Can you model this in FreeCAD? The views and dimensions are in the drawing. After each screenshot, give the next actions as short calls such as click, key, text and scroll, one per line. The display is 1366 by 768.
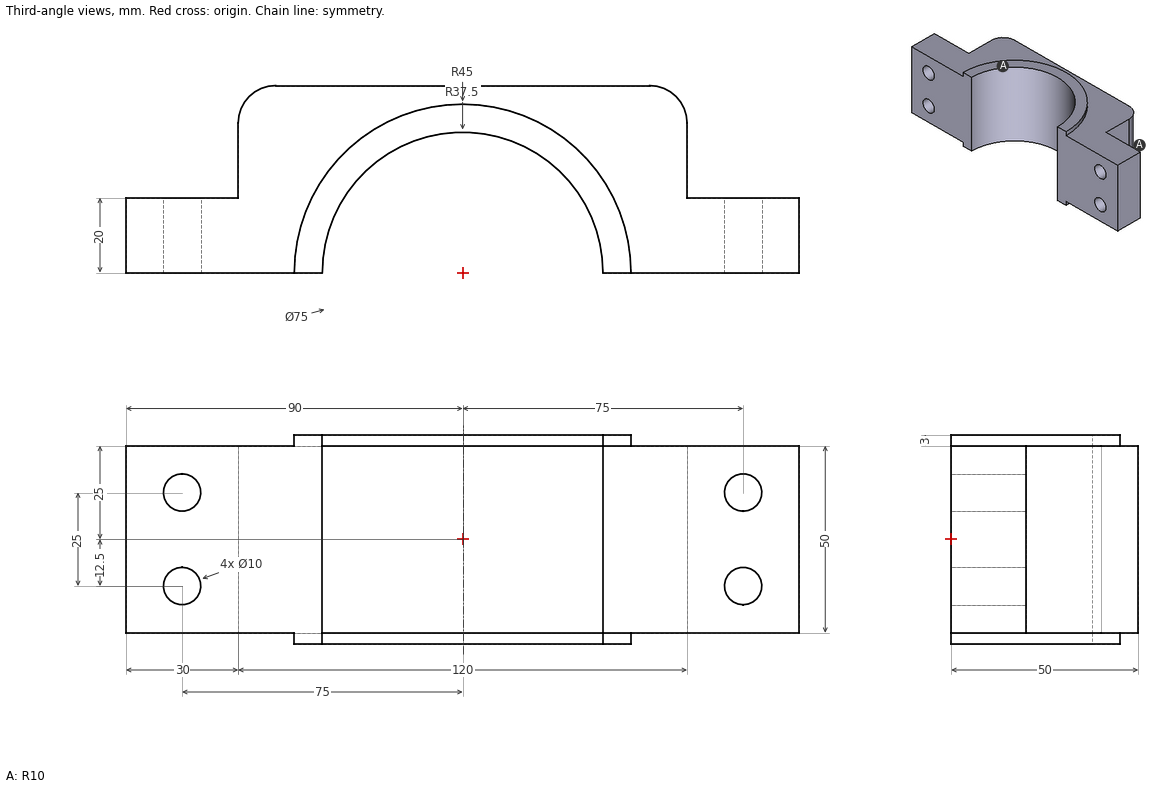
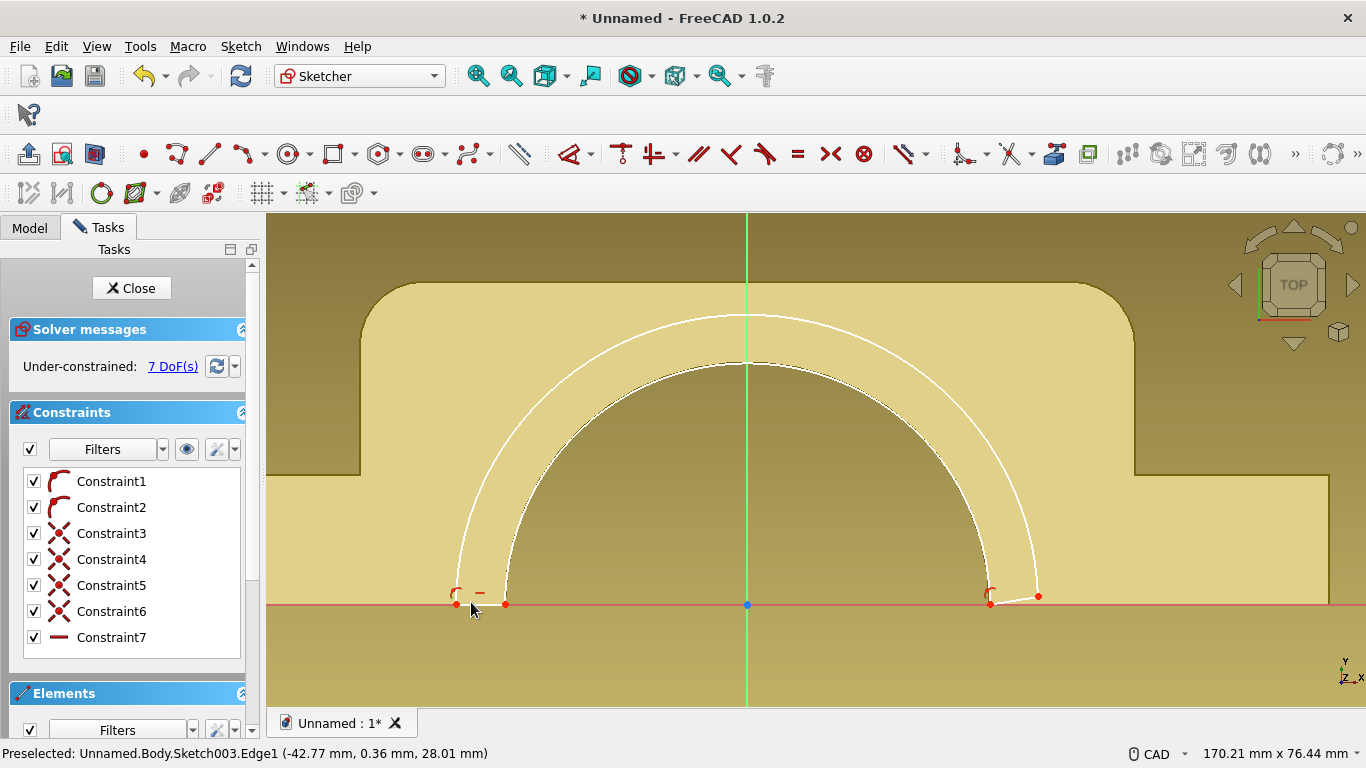
click(1004, 602)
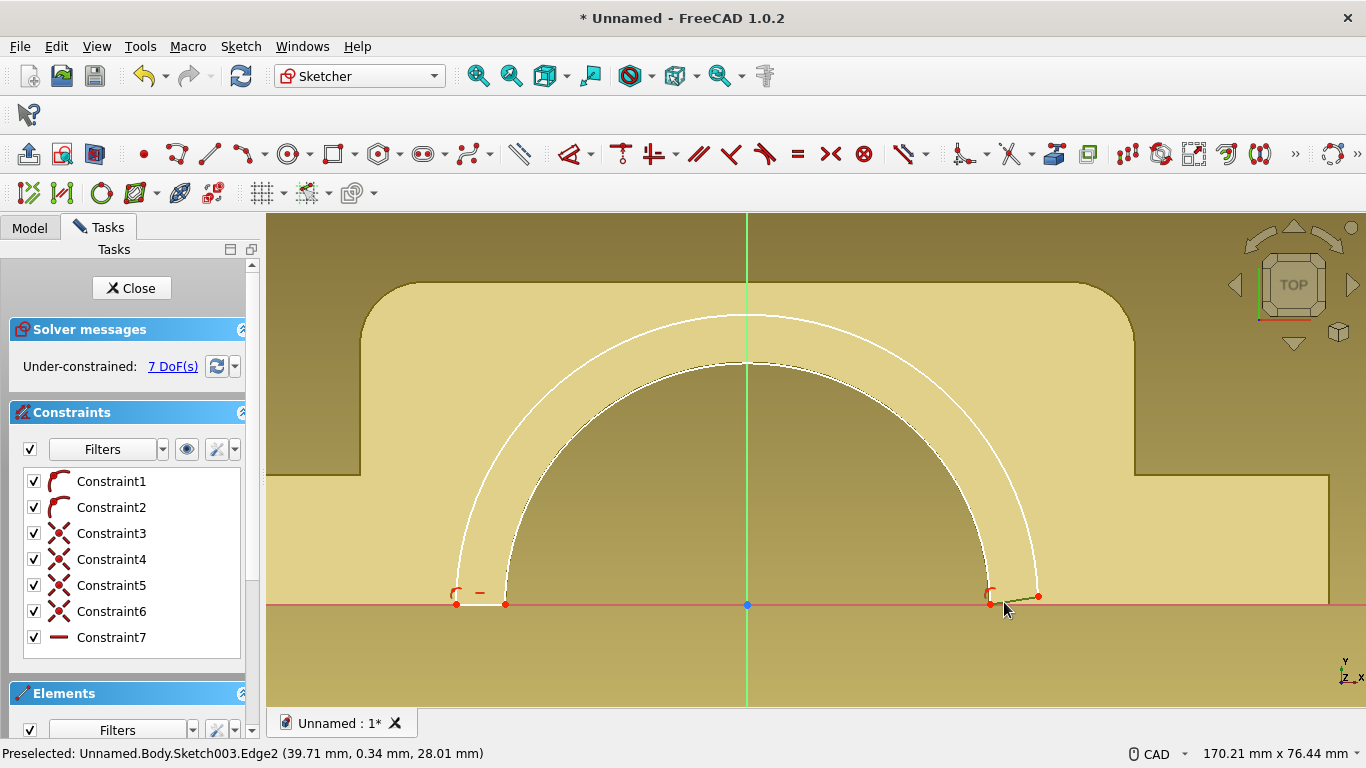
key(h)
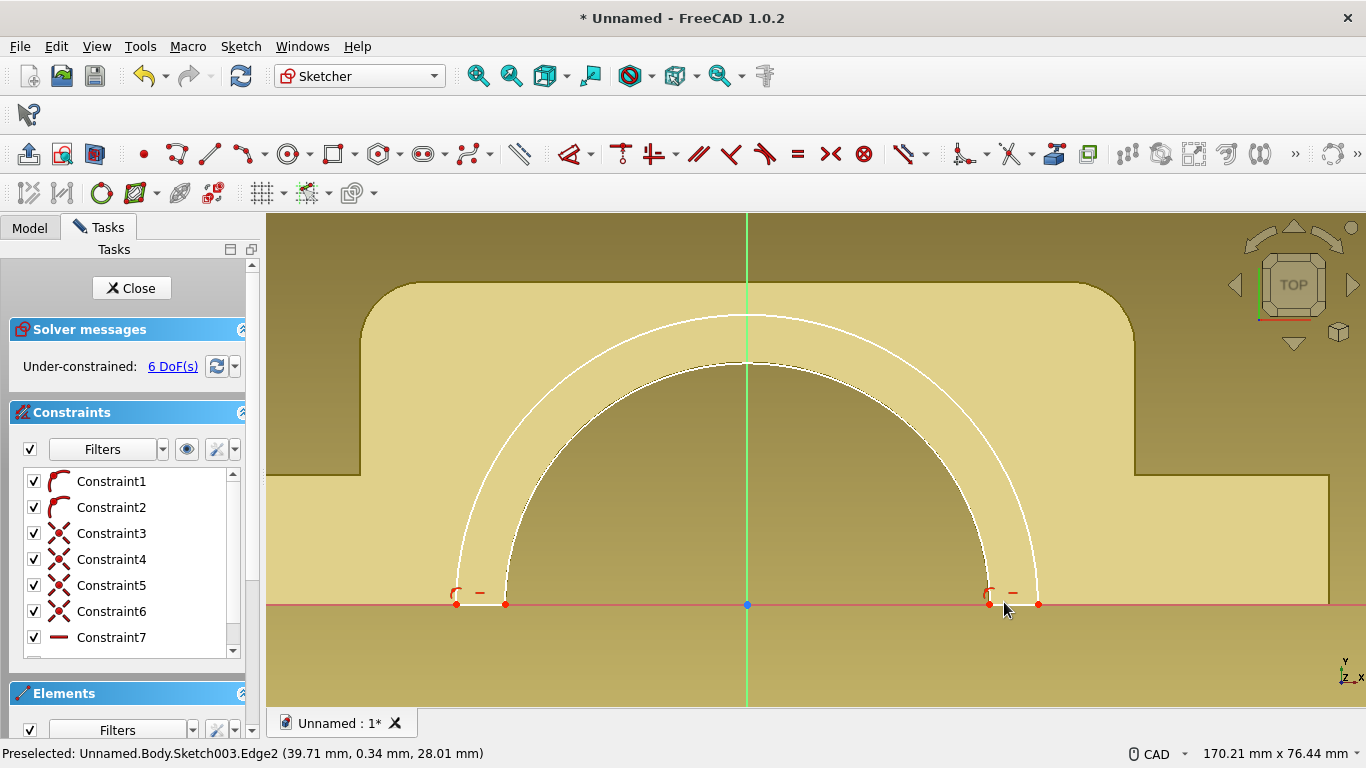
click(890, 409)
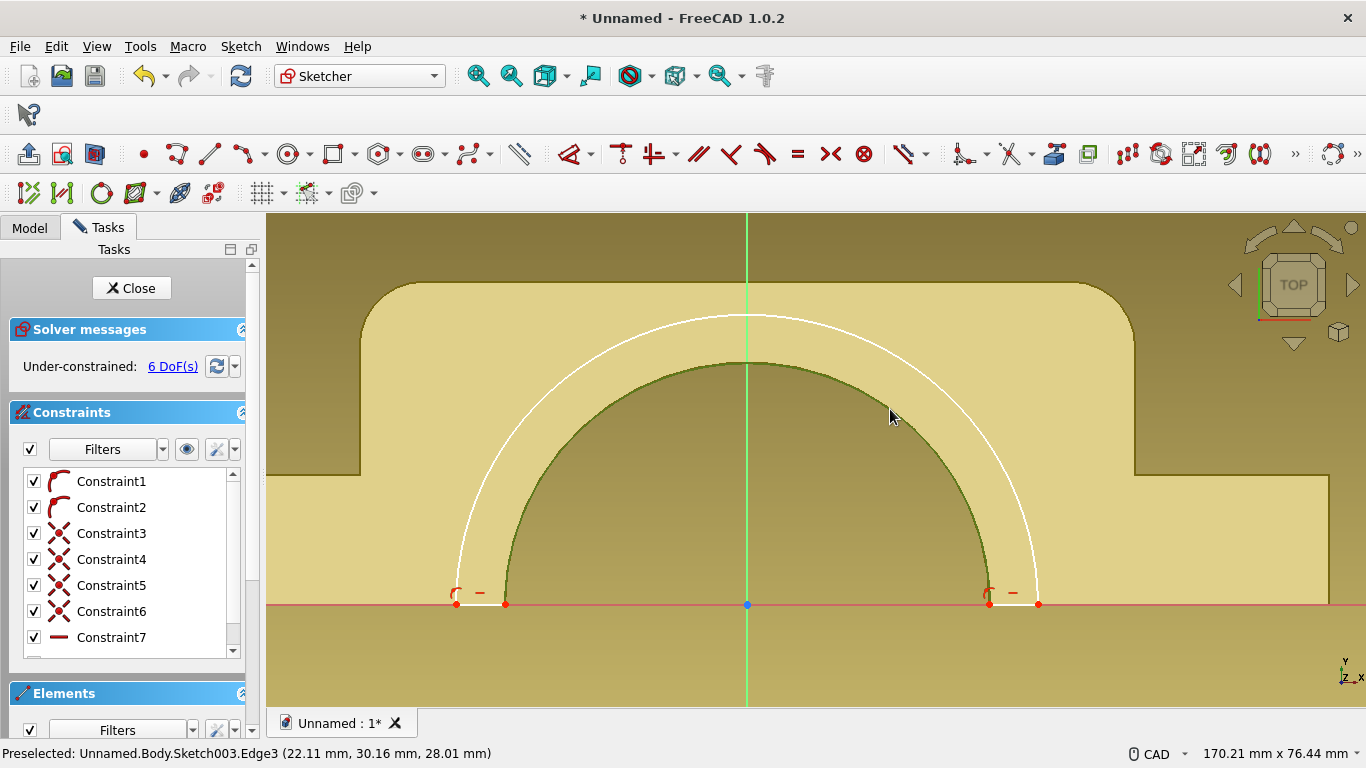
click(918, 370)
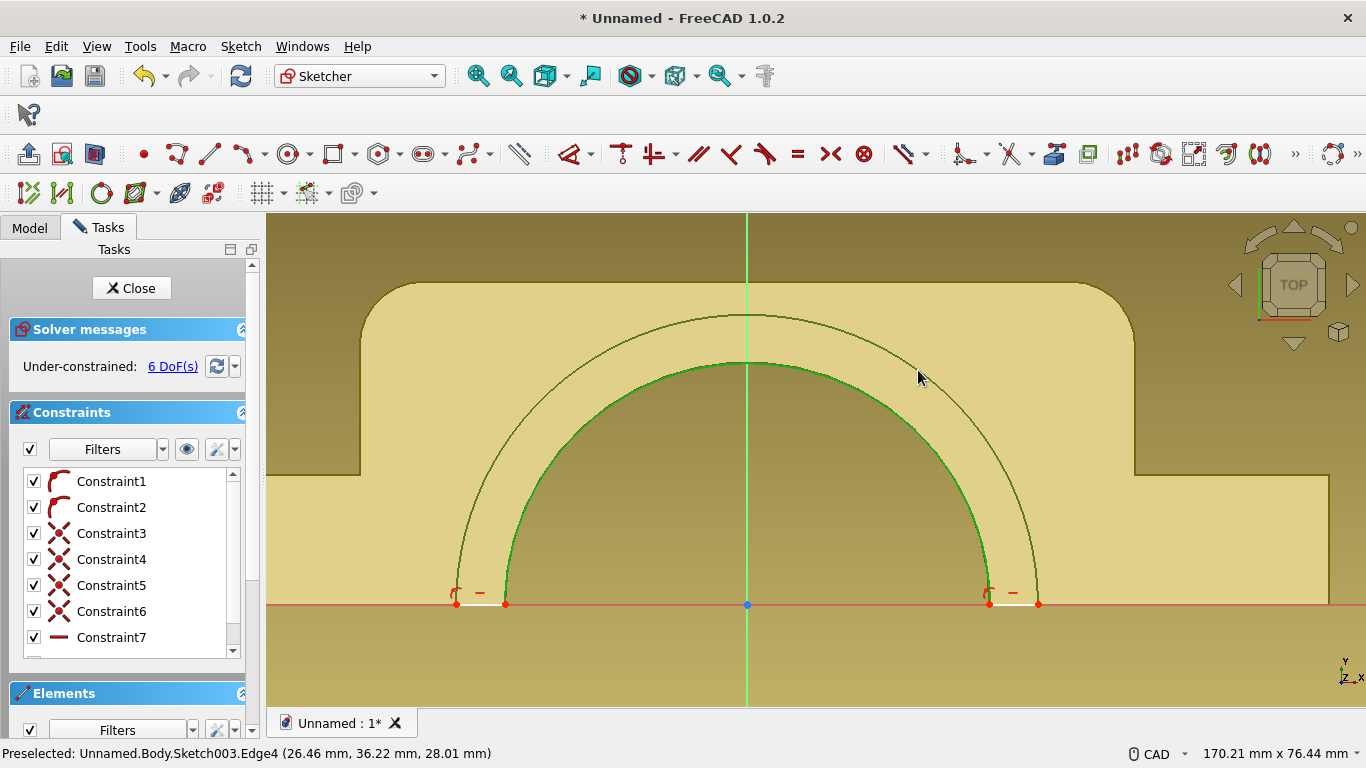
key(c)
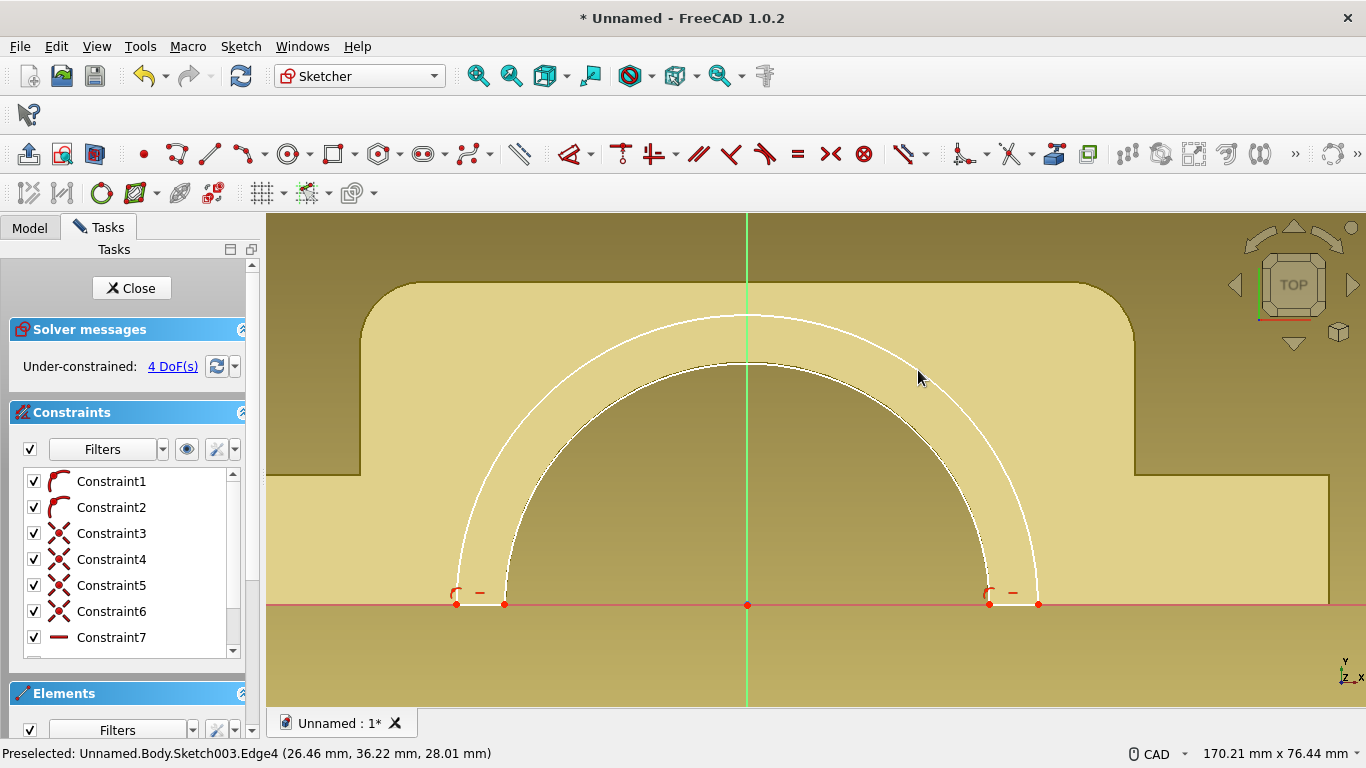
drag(737, 595, 757, 616)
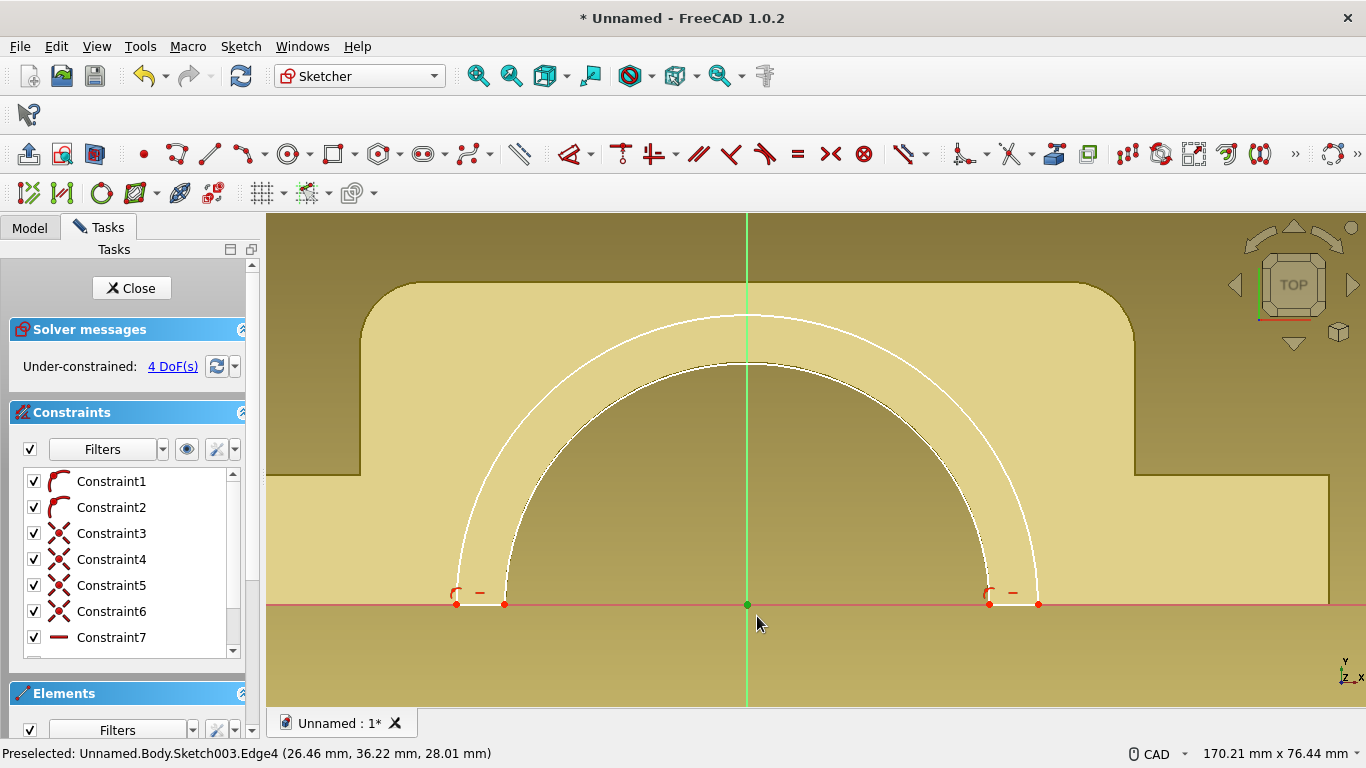
key(c)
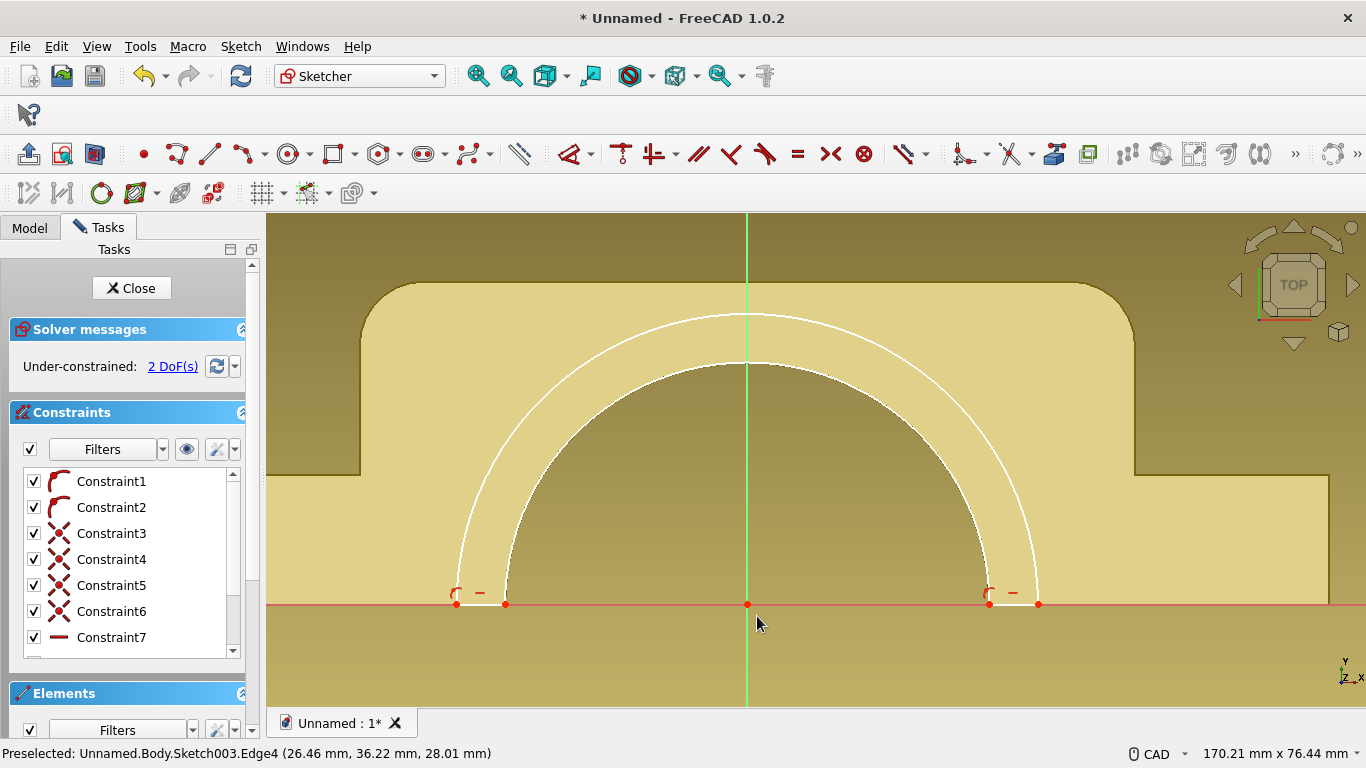
click(890, 409)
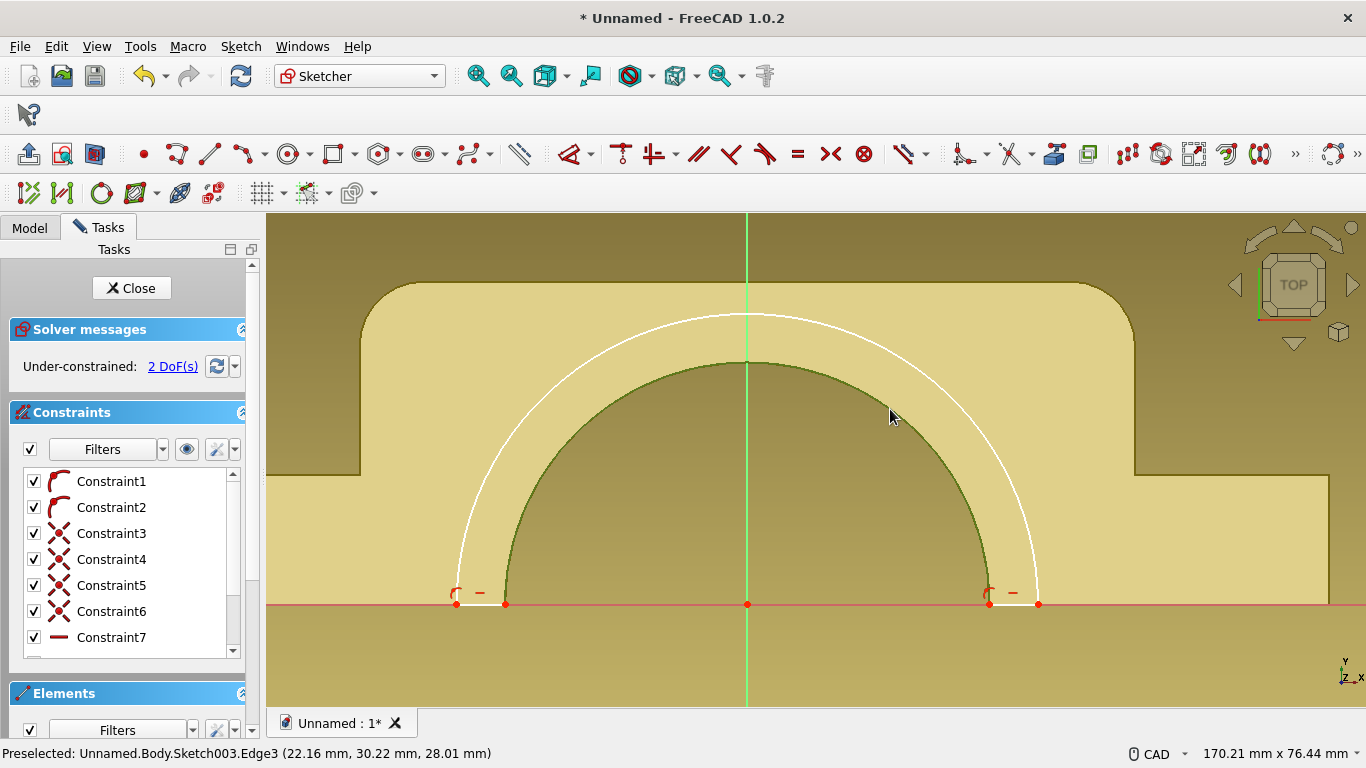
key(k)
key(r)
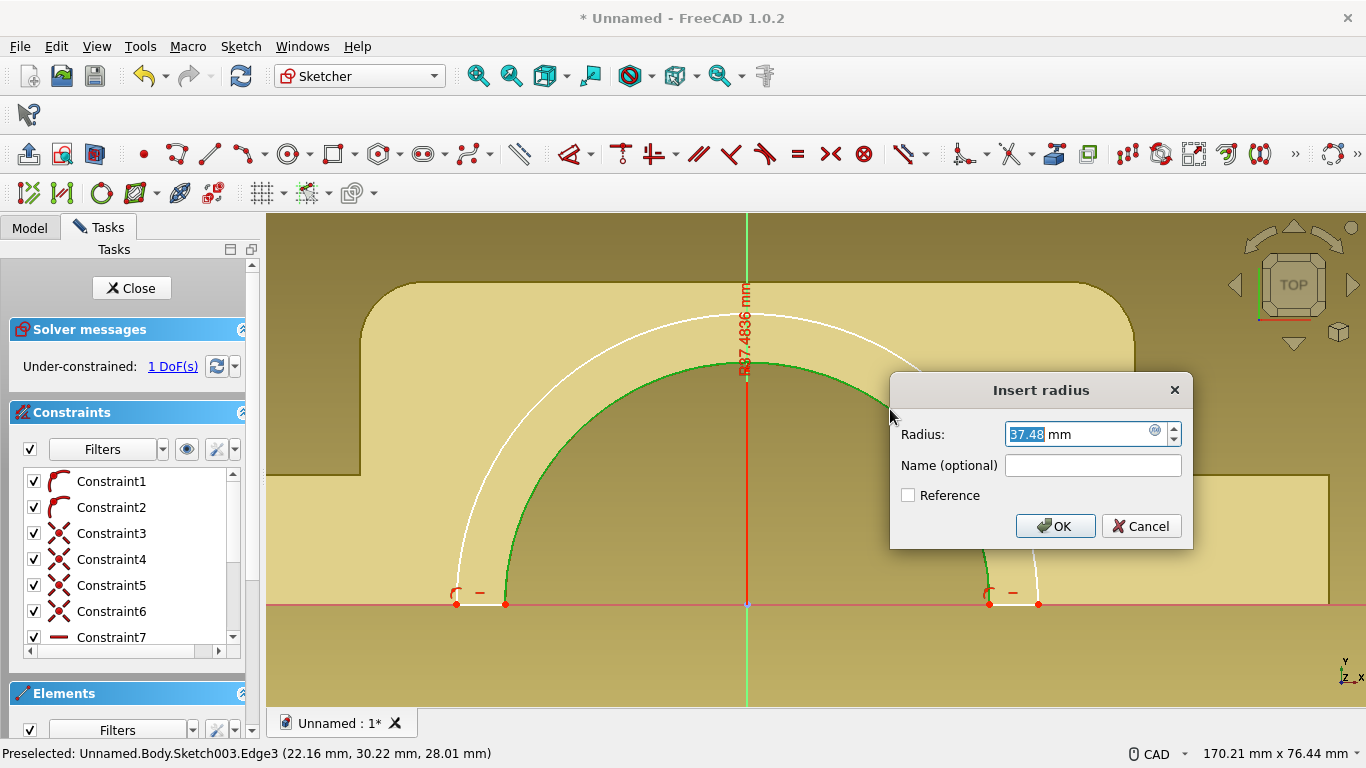
text(37.5)
key(Return)